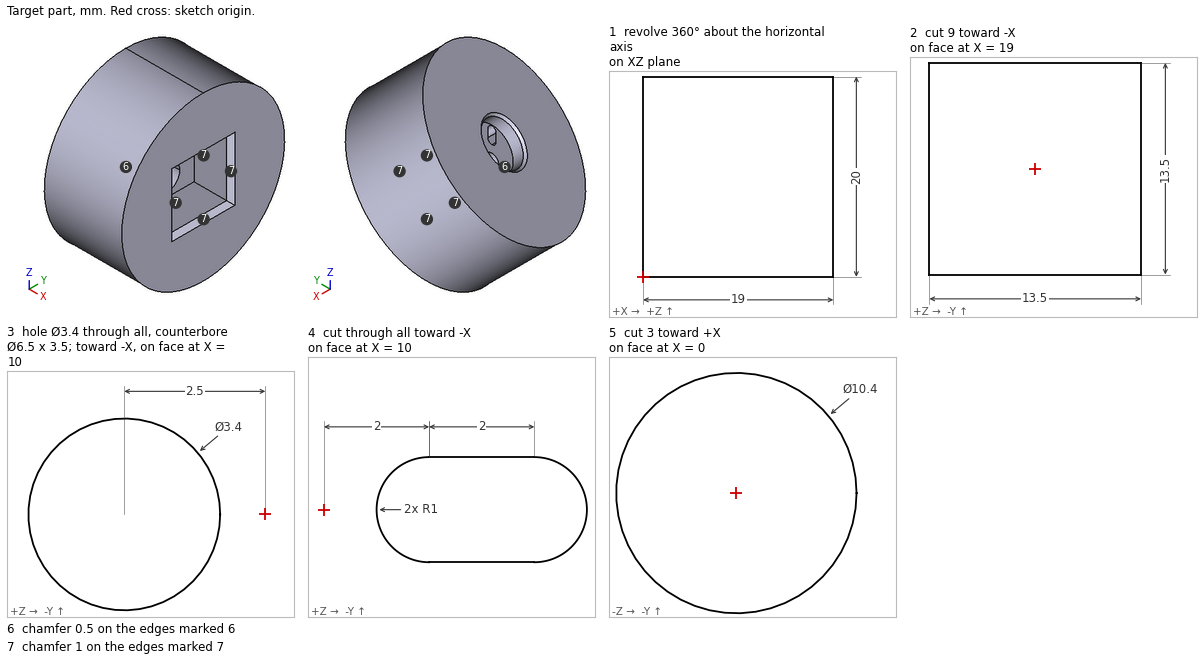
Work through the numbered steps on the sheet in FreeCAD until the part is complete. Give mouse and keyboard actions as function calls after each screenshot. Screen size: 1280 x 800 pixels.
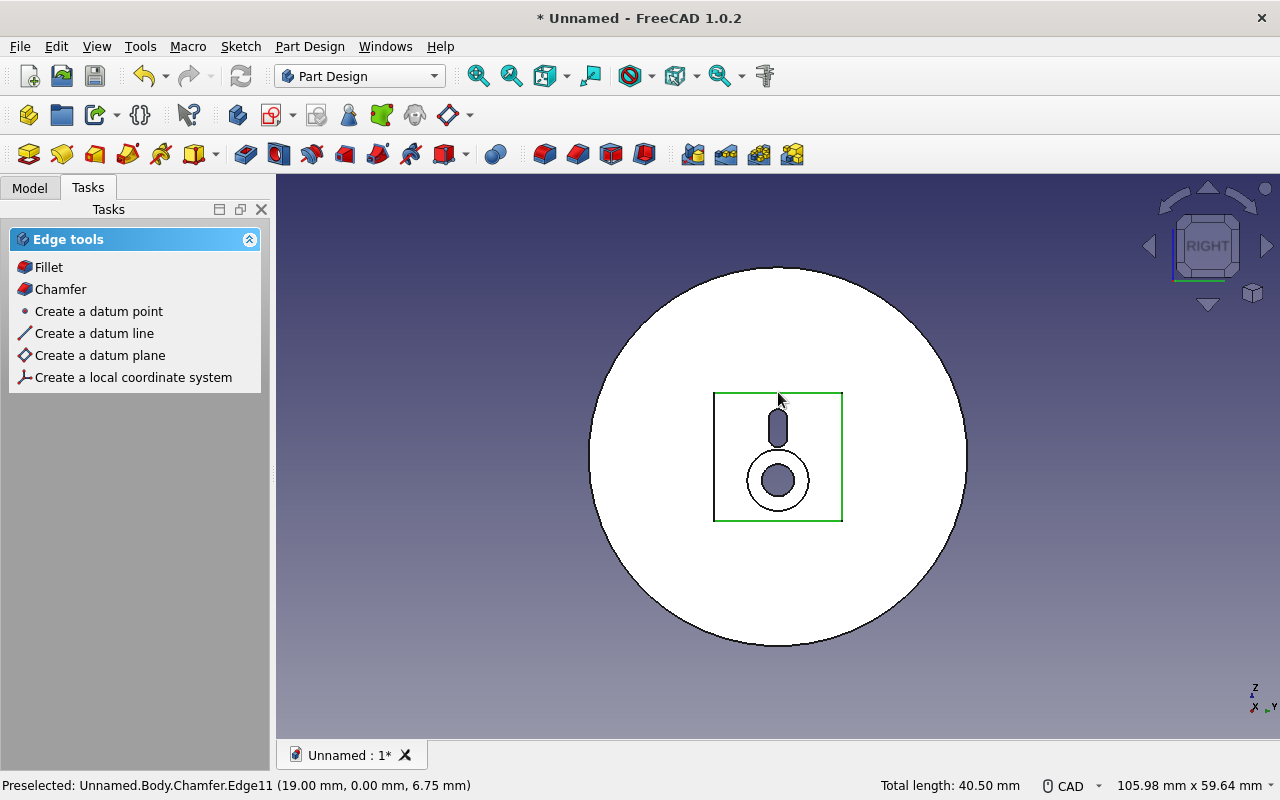
click(714, 456, ctrl)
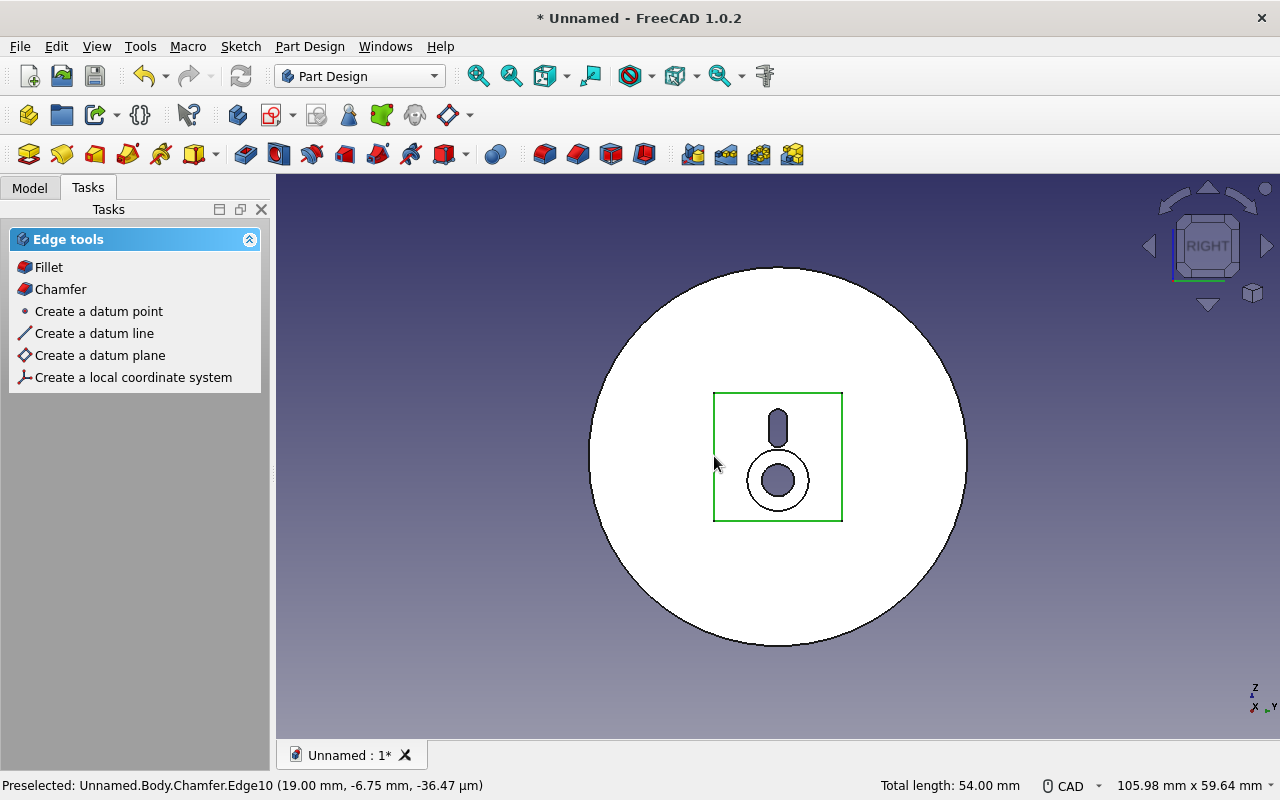
click(578, 154)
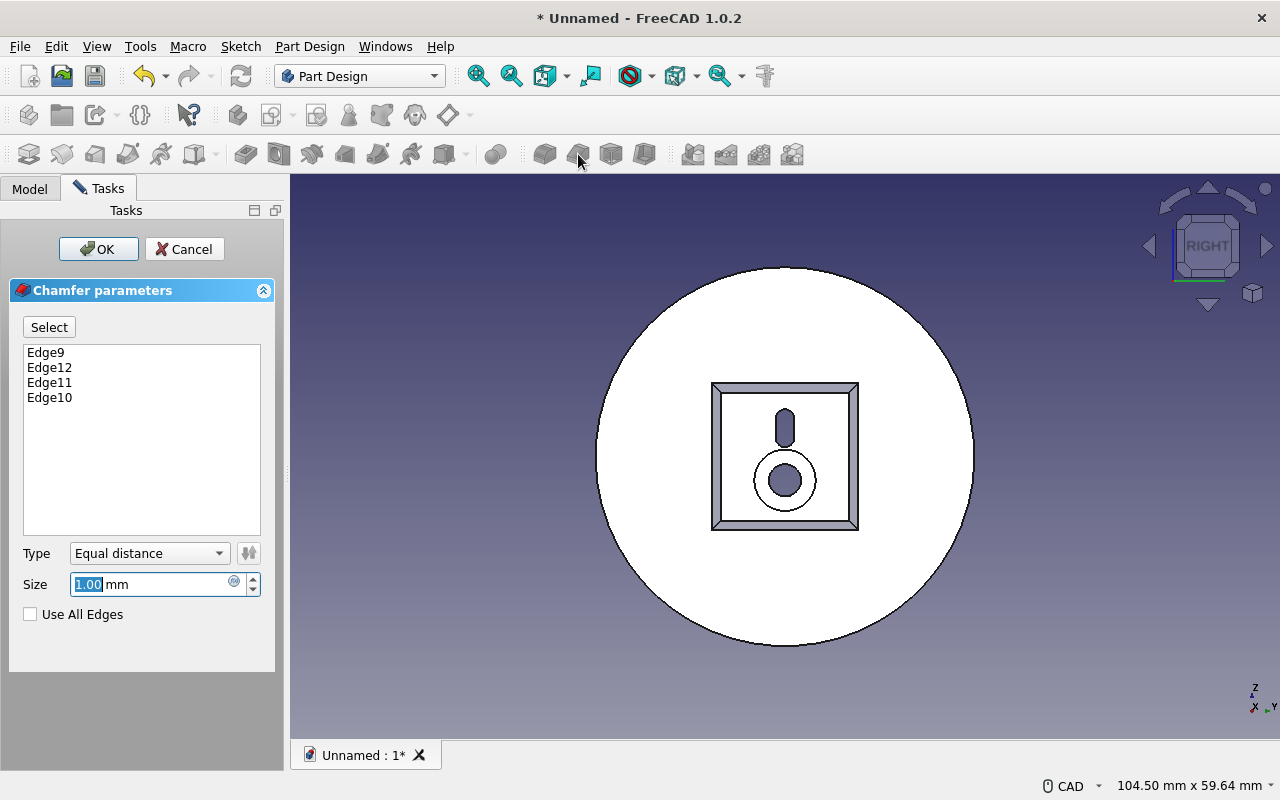
text(1)
key(Tab)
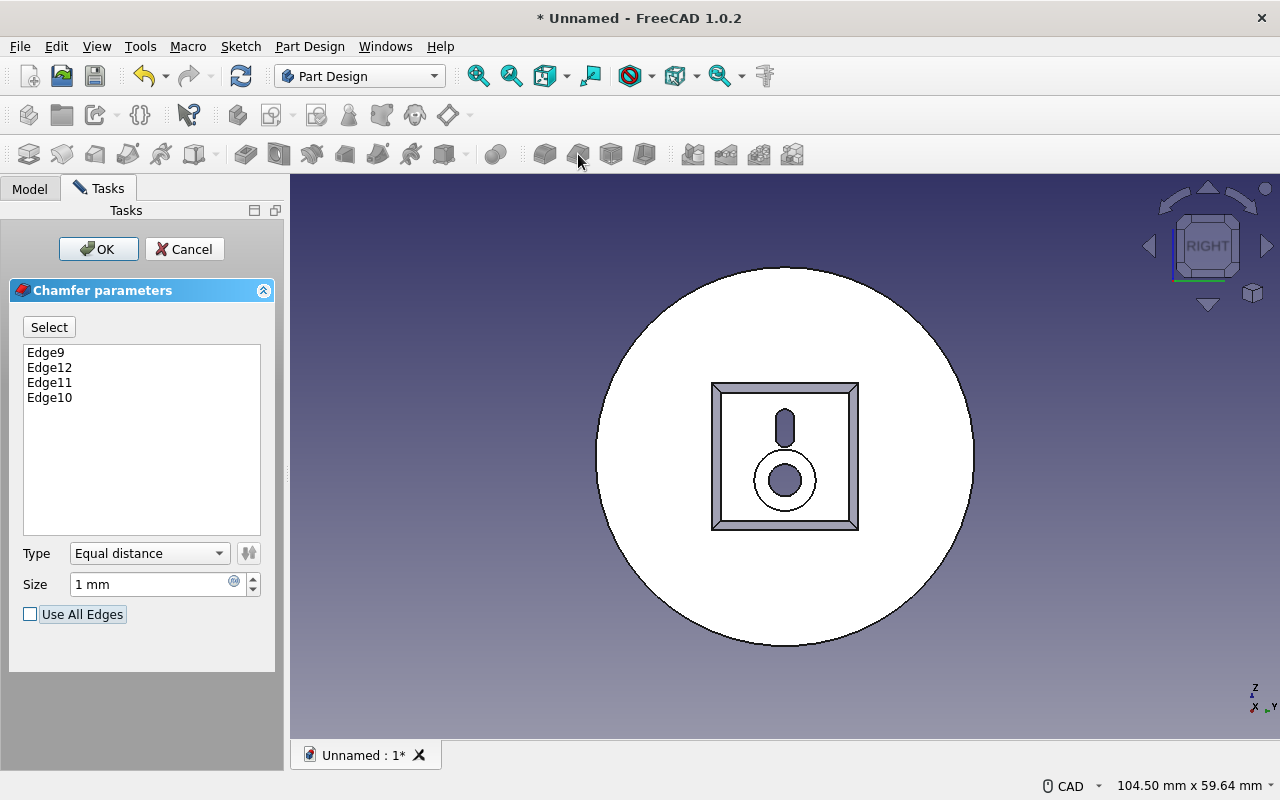
click(99, 249)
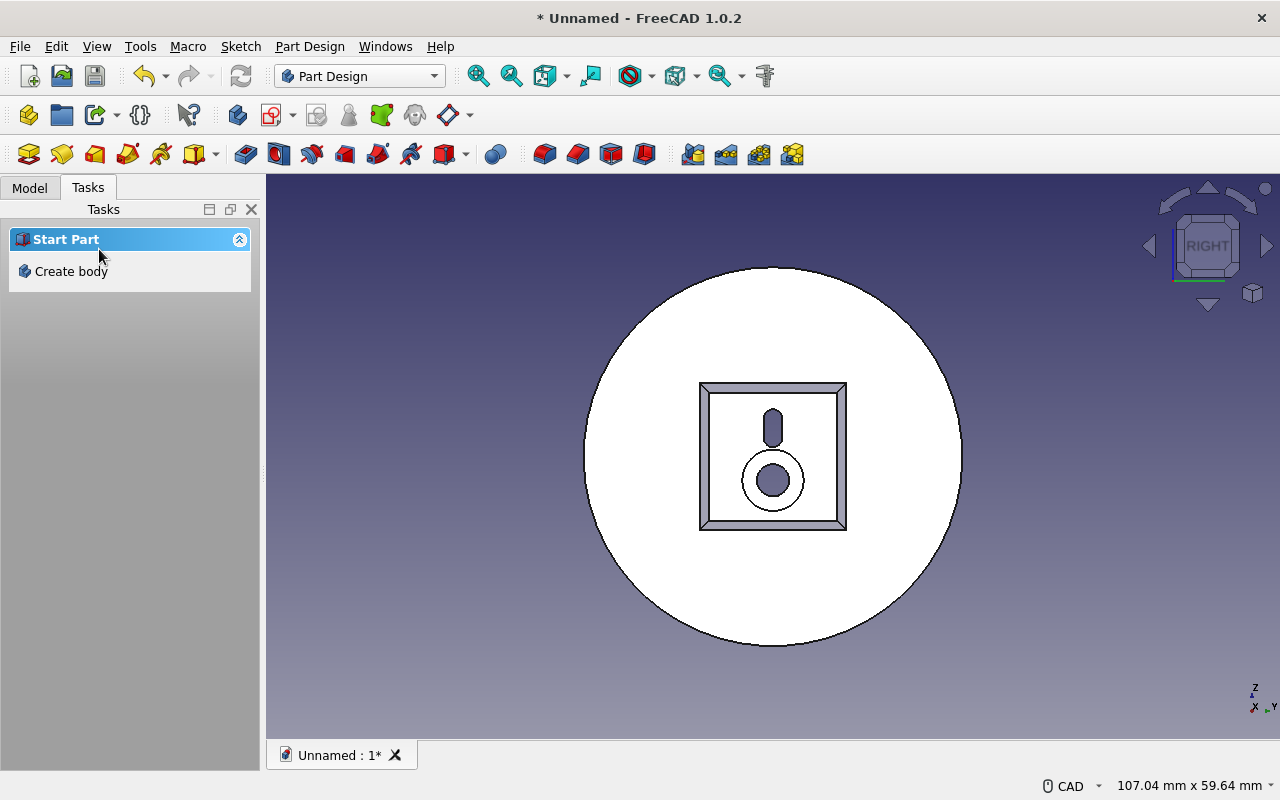
key(0)